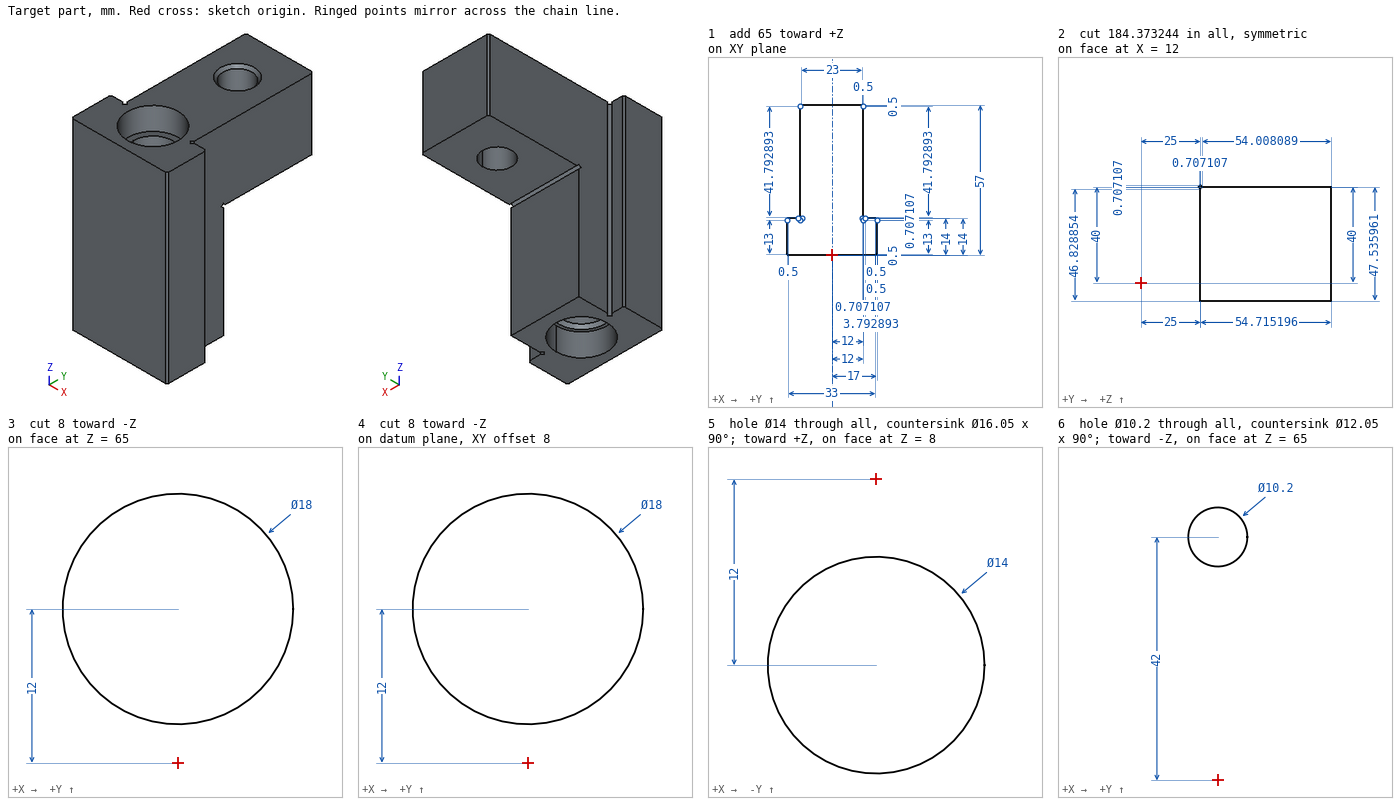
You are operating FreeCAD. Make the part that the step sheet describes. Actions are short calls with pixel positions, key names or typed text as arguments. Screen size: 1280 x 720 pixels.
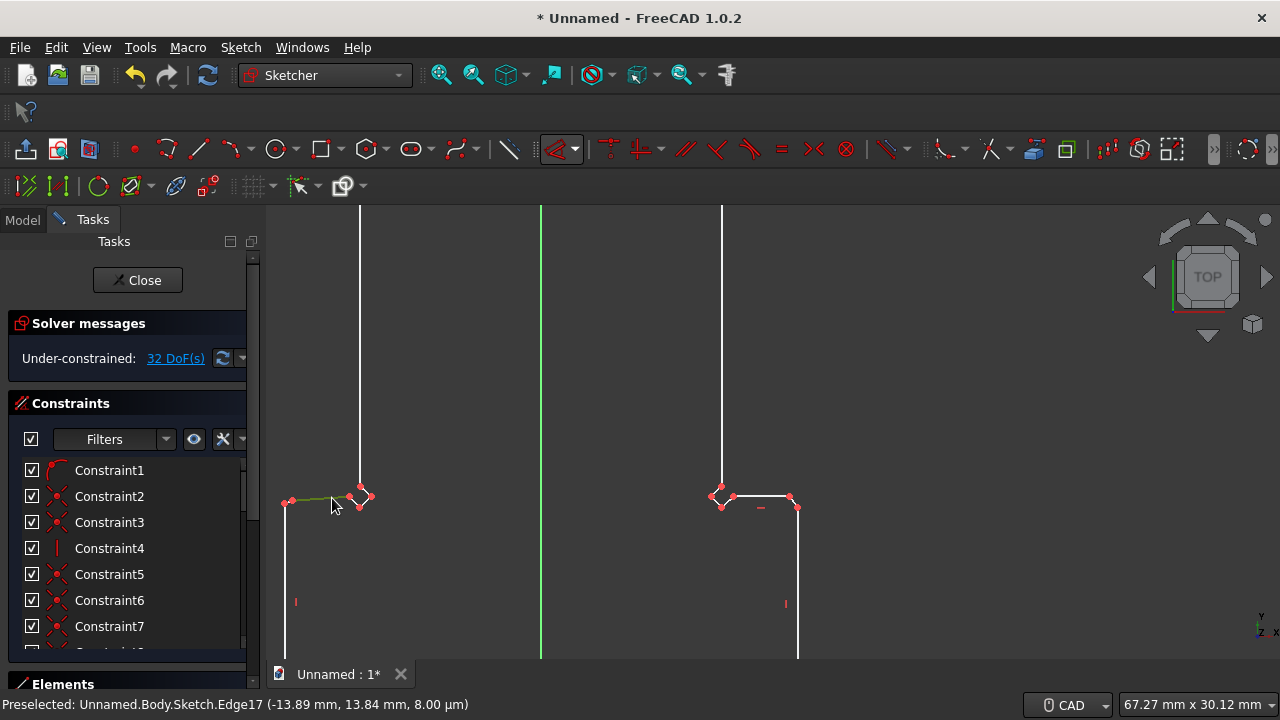
key(h)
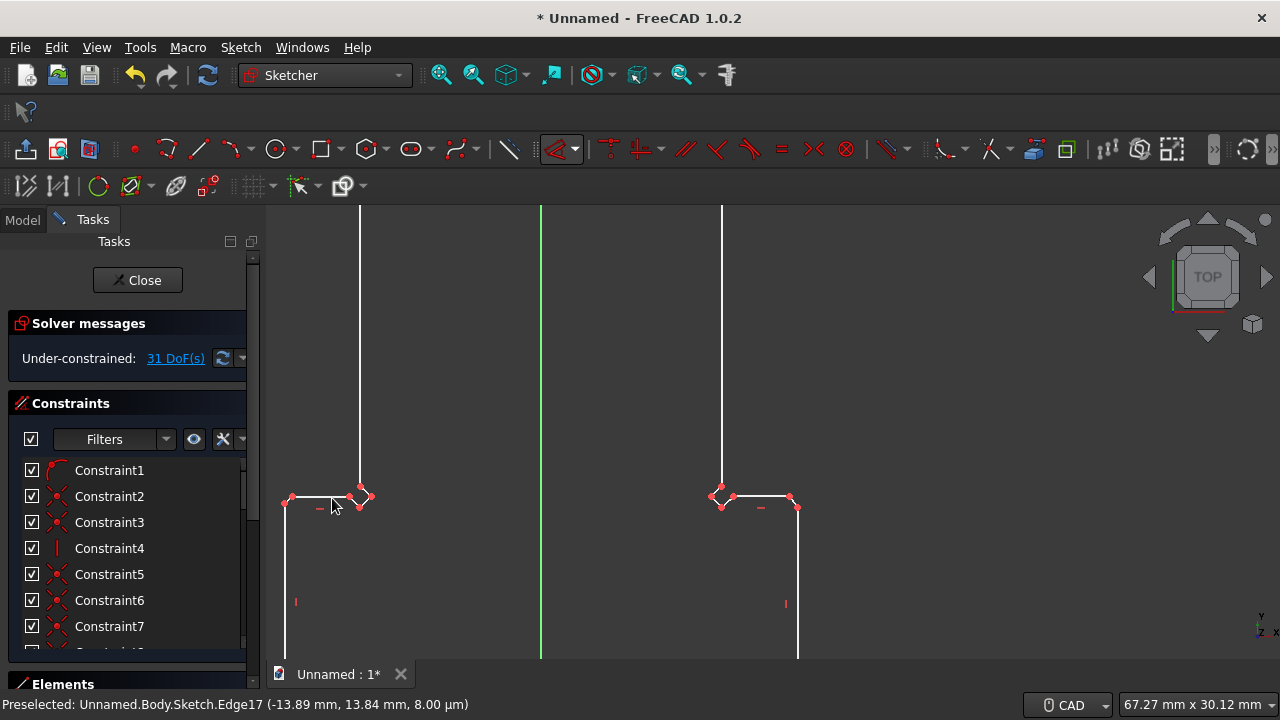
scroll(775, 499, down, 6)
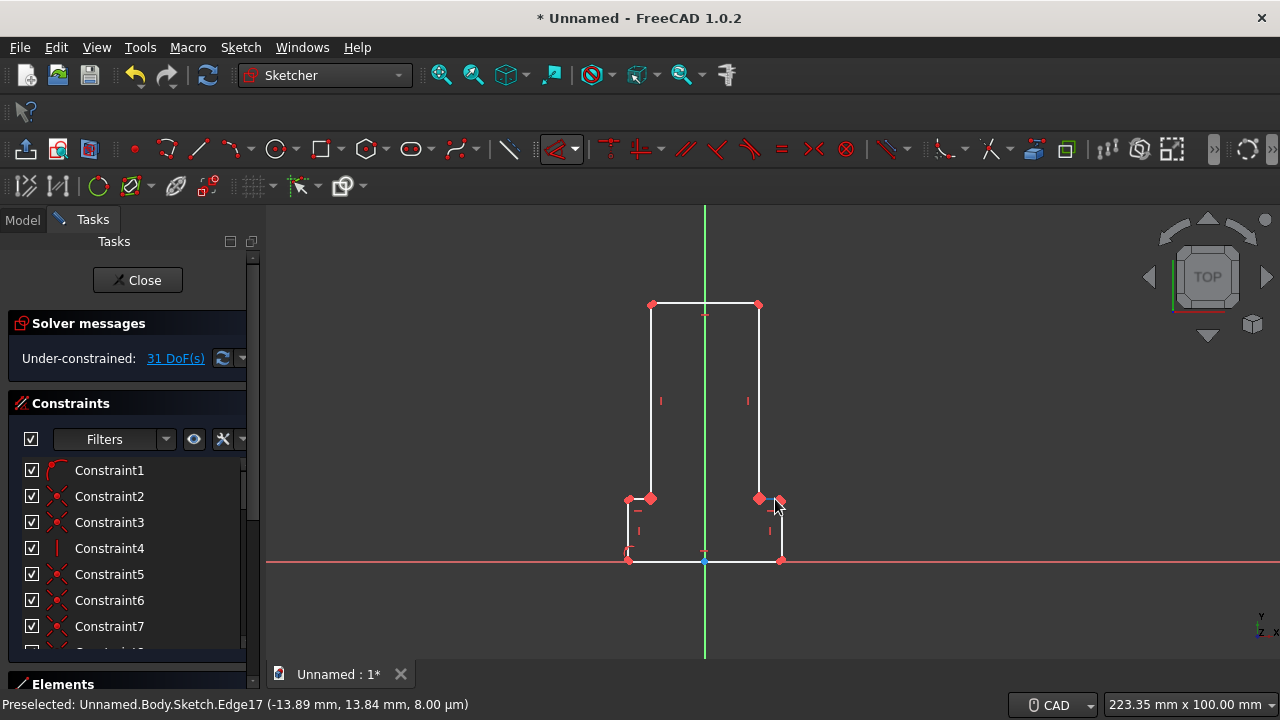
scroll(759, 306, up, 7)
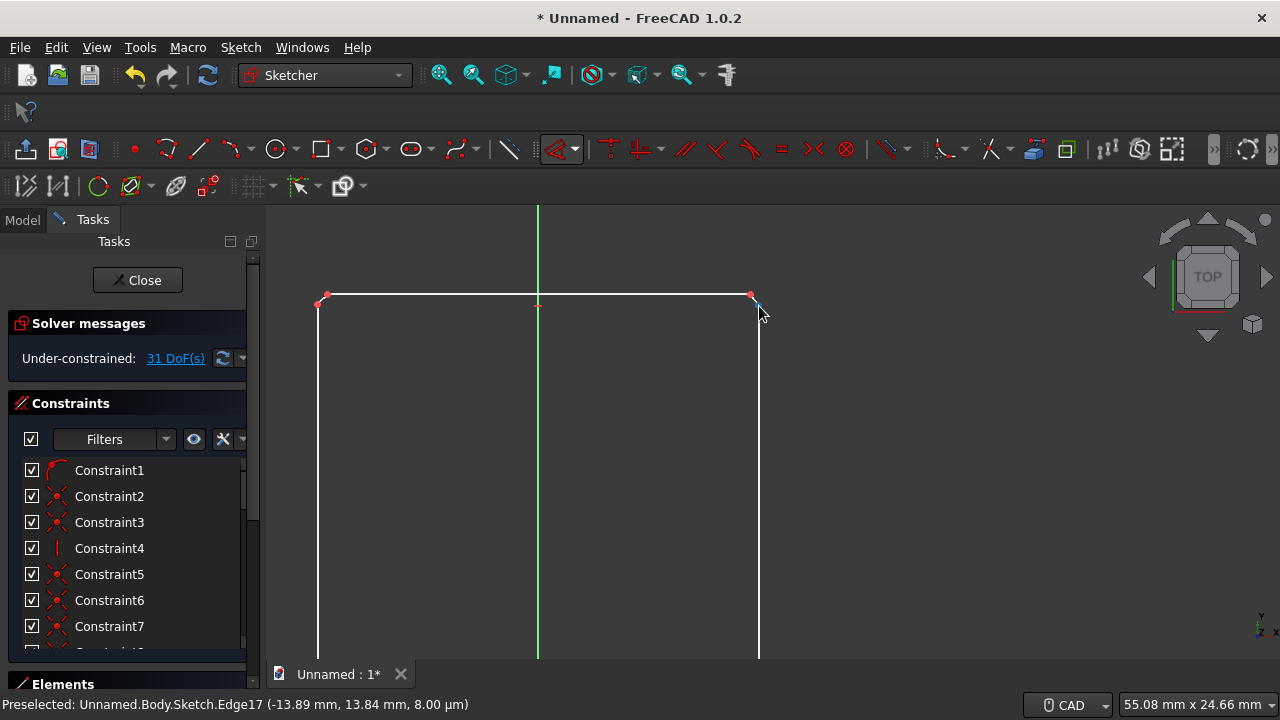
click(759, 305)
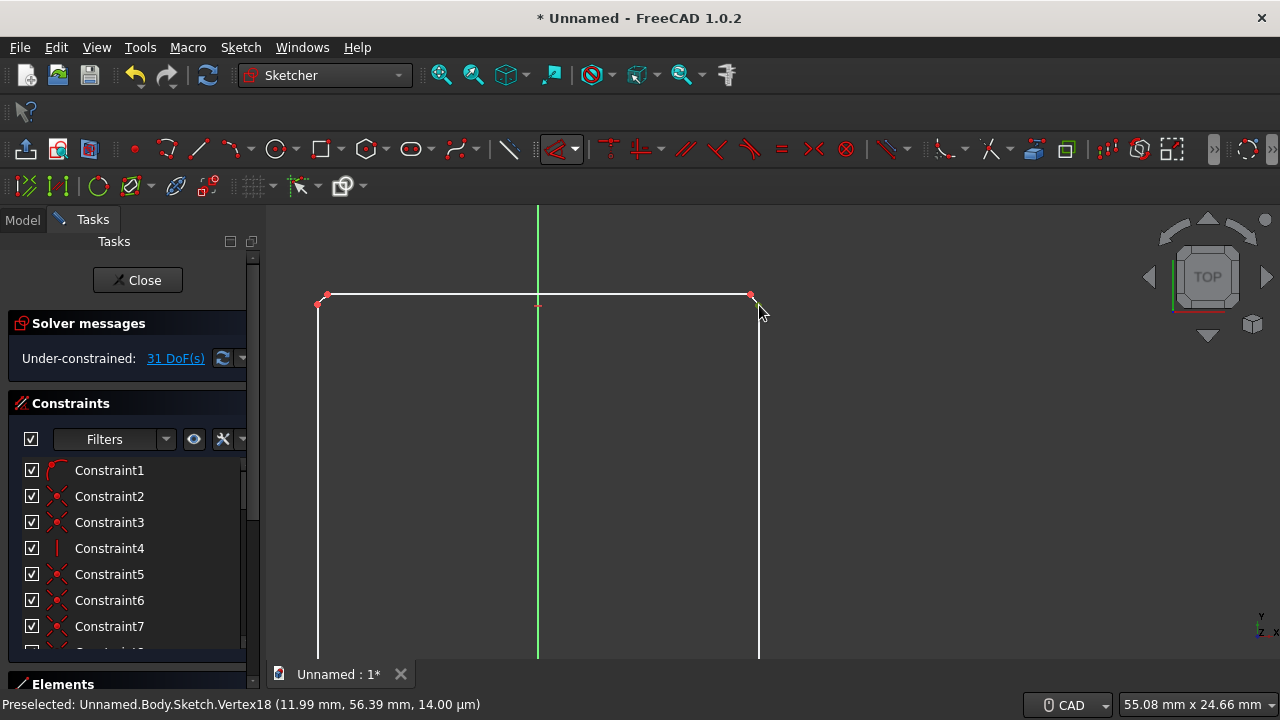
click(318, 304)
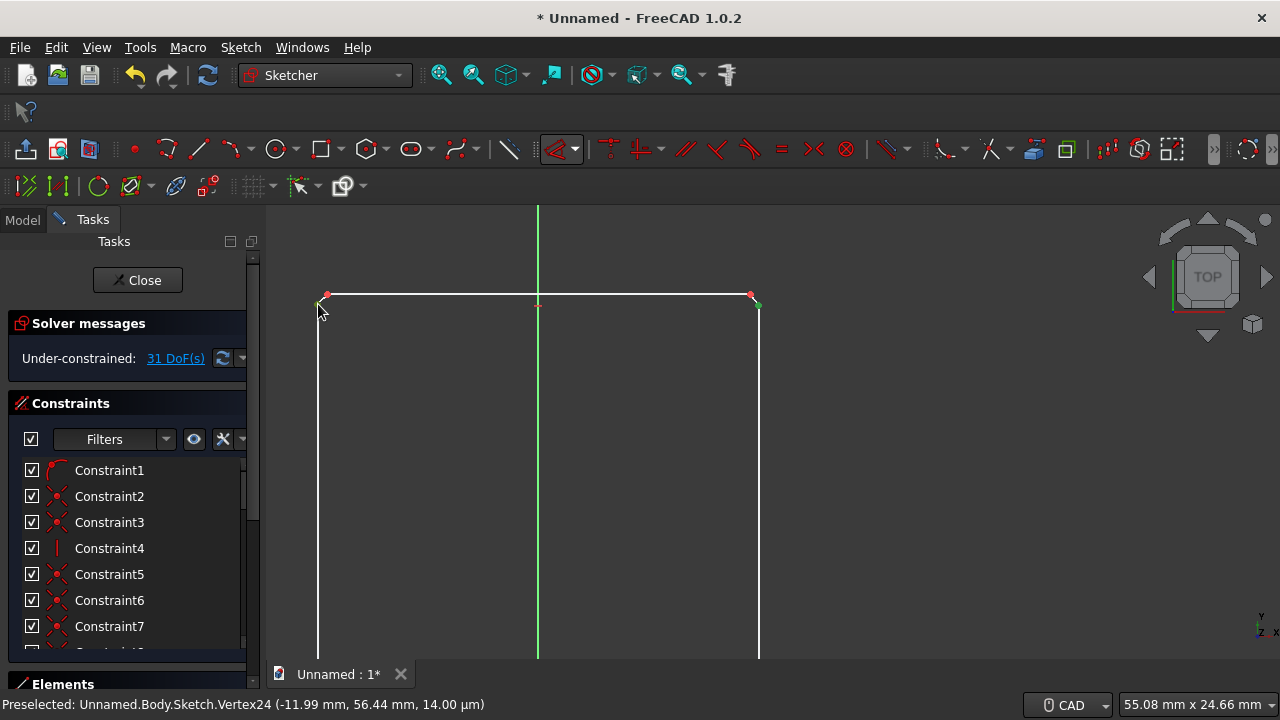
click(538, 603)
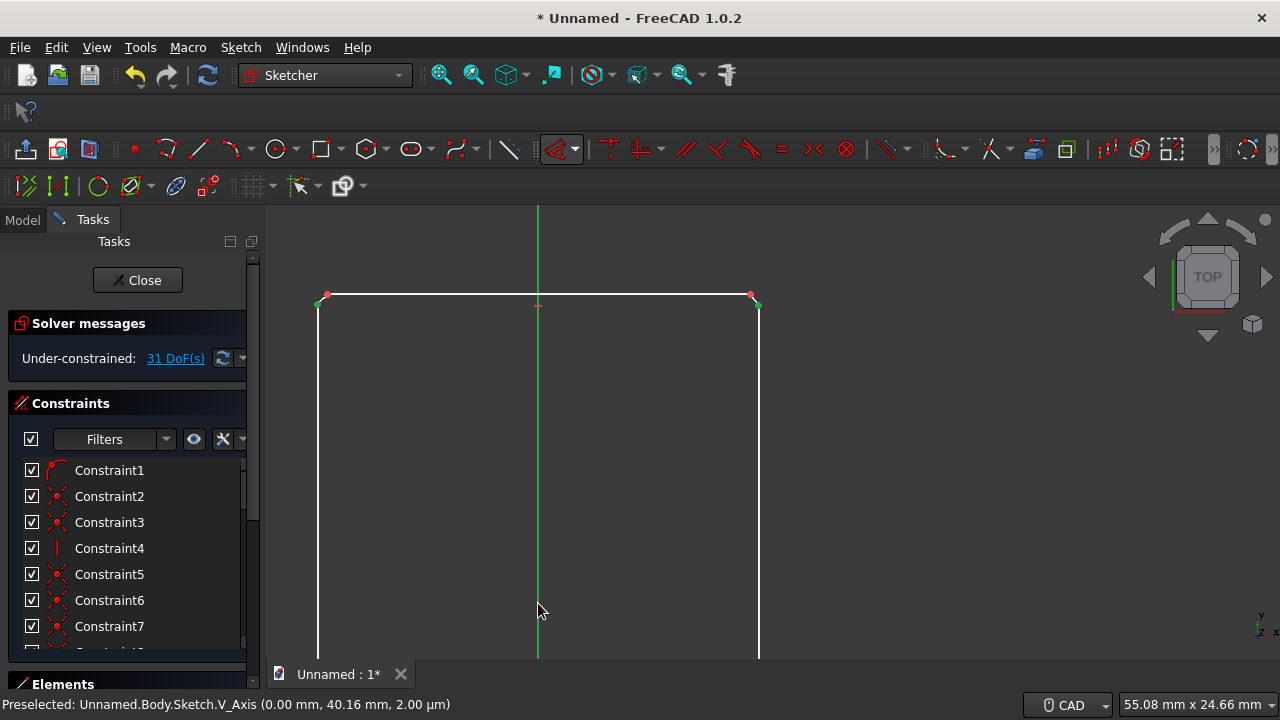
key(s)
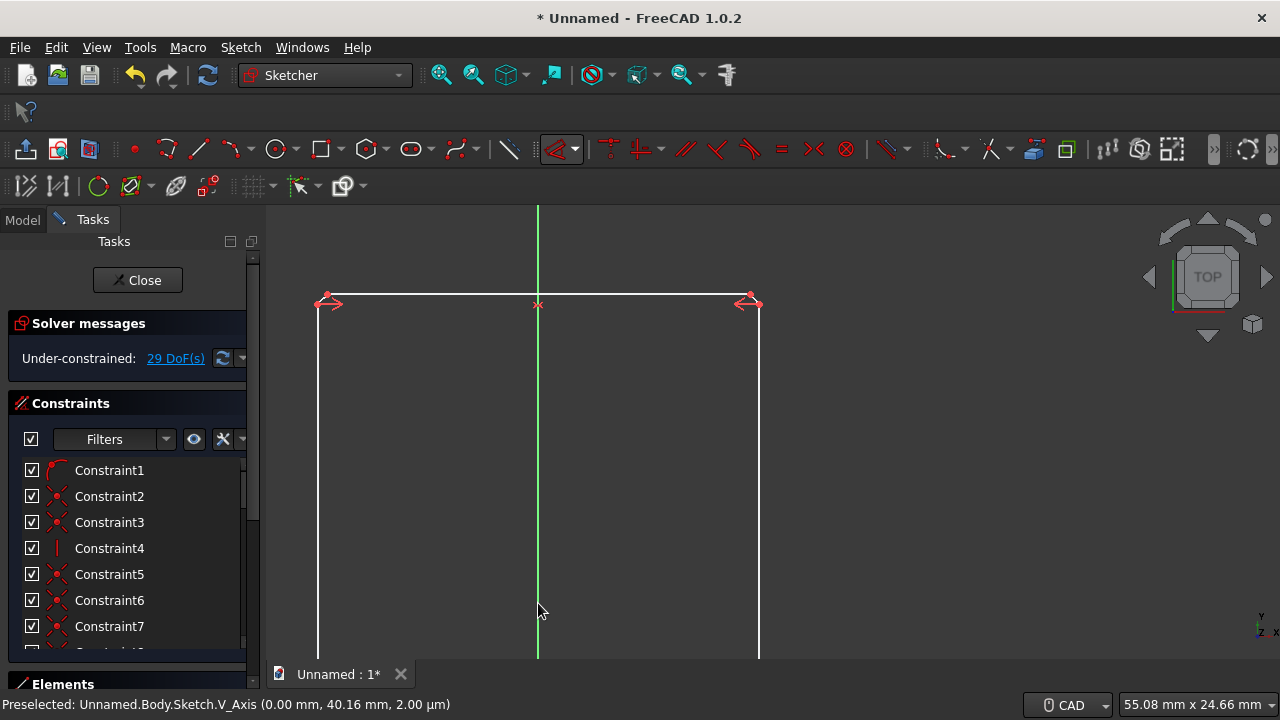
scroll(759, 305, down, 7)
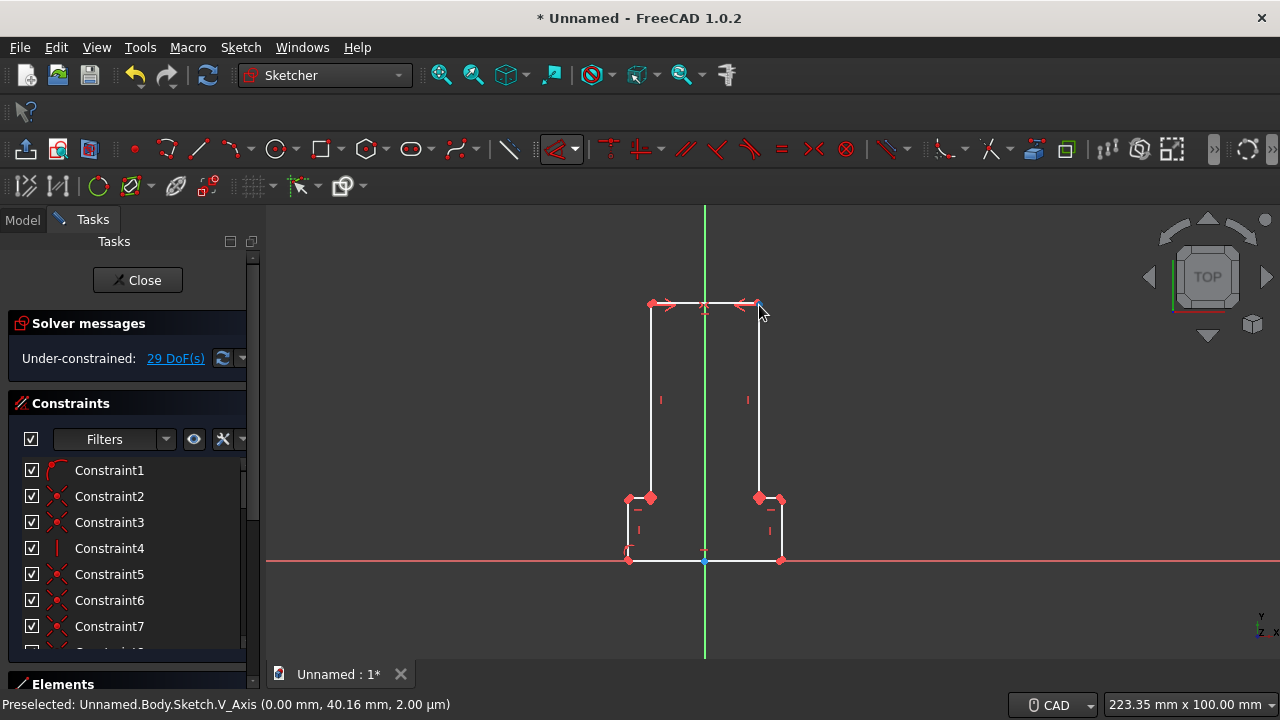
scroll(756, 498, up, 5)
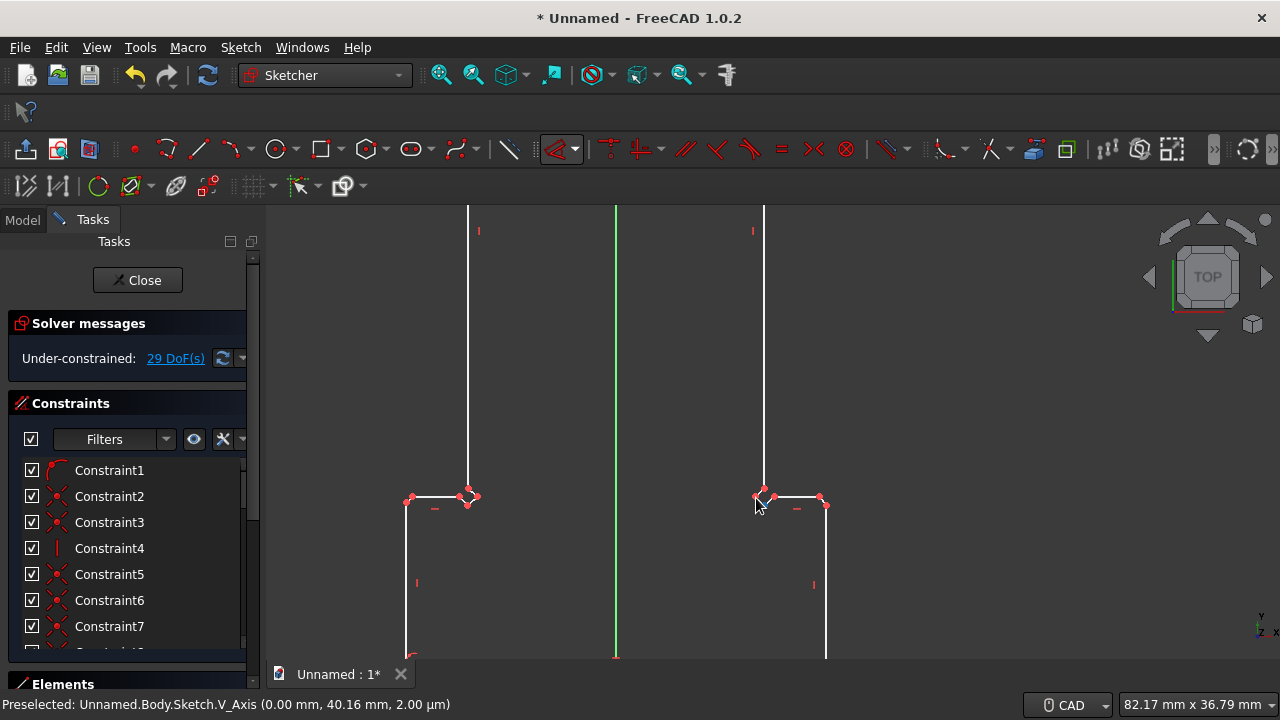
click(756, 497)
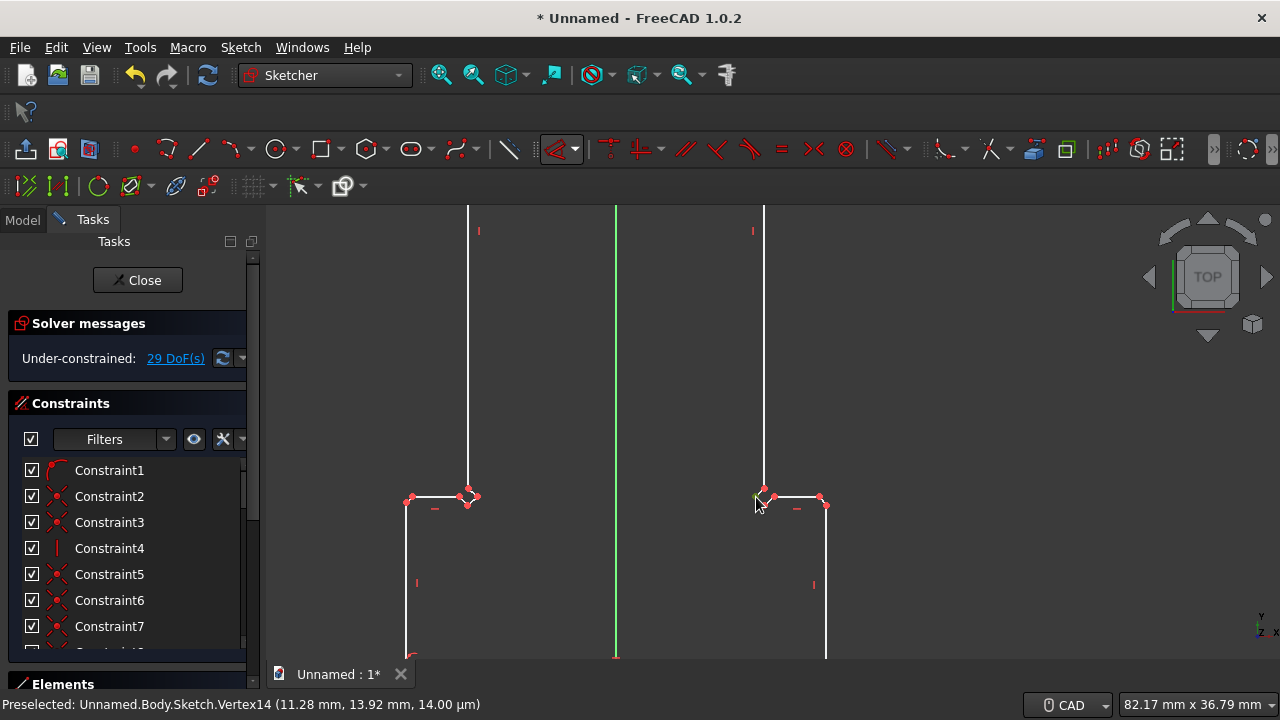
click(477, 497)